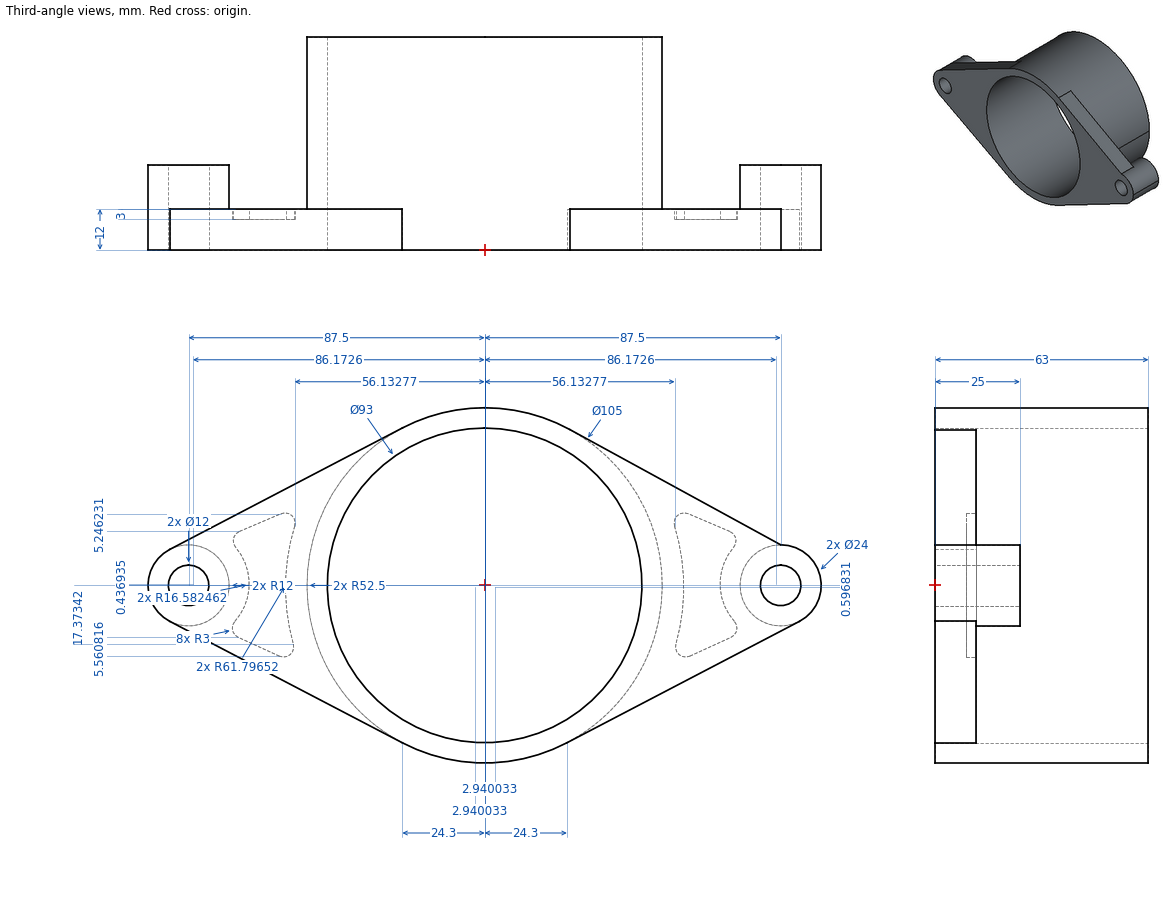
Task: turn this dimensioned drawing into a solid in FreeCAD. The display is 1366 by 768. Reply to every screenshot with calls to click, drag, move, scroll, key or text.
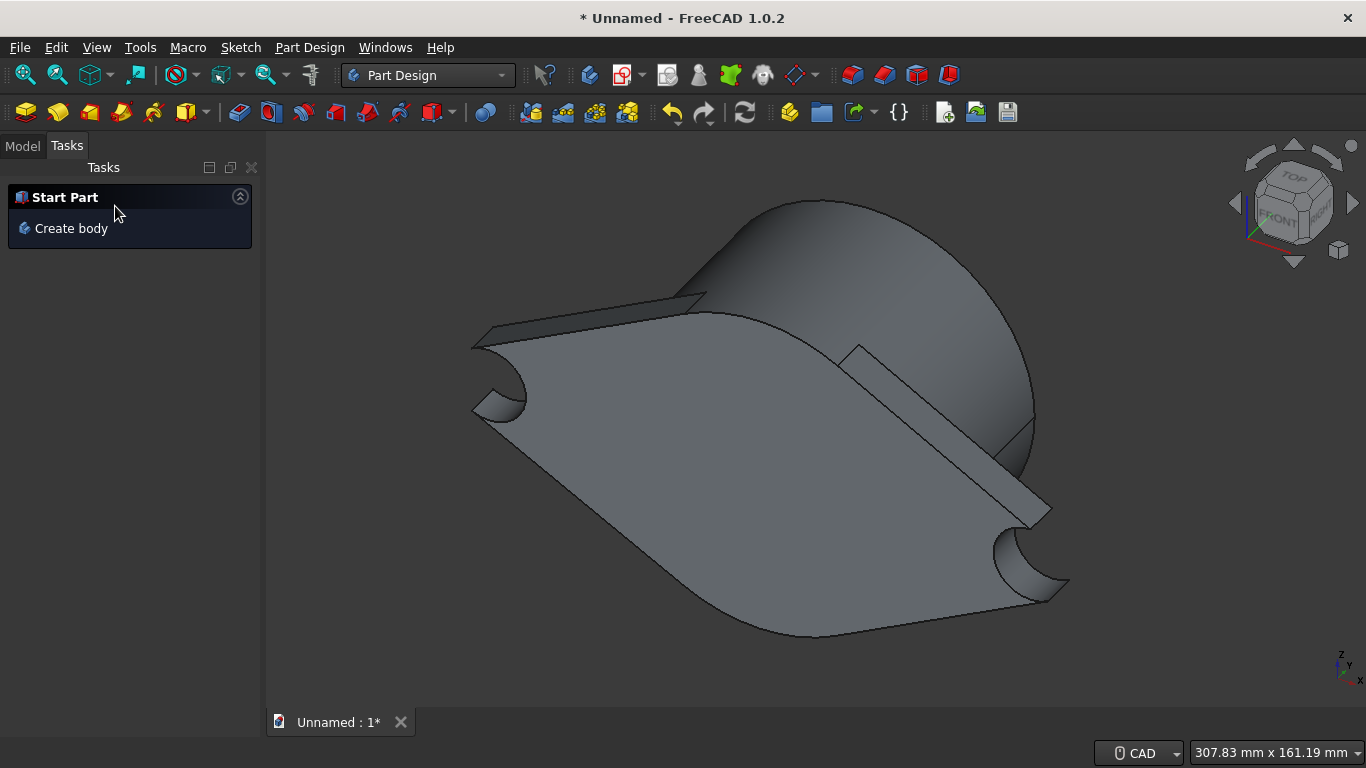
key(v)
key(f)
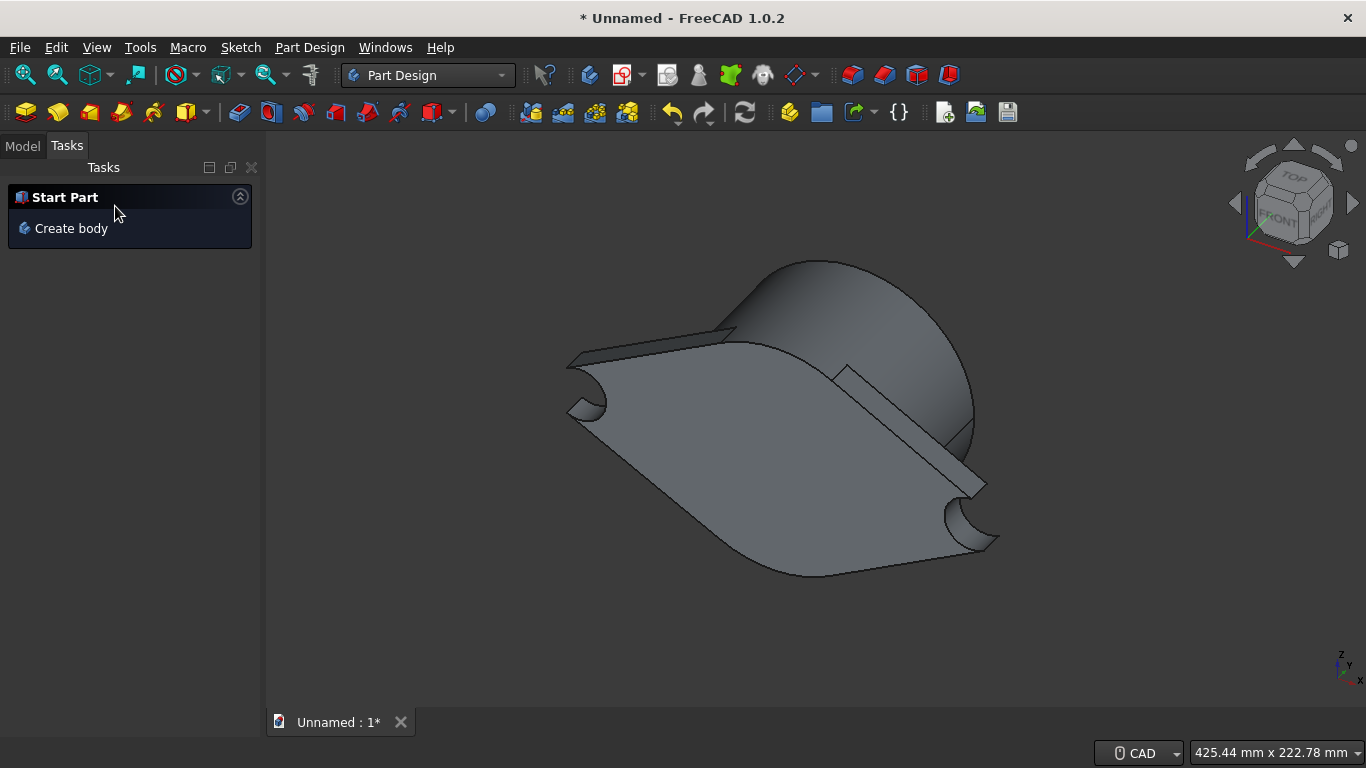
click(775, 458)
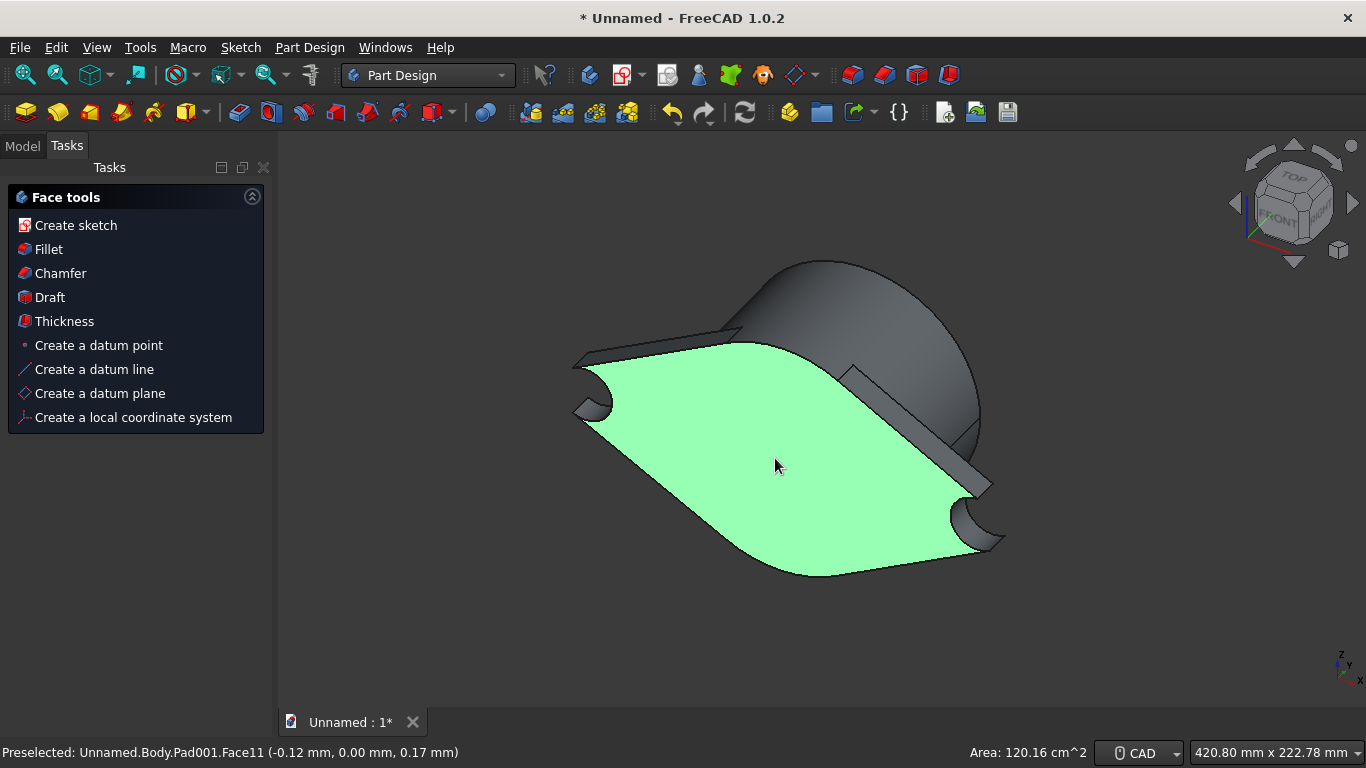
click(622, 76)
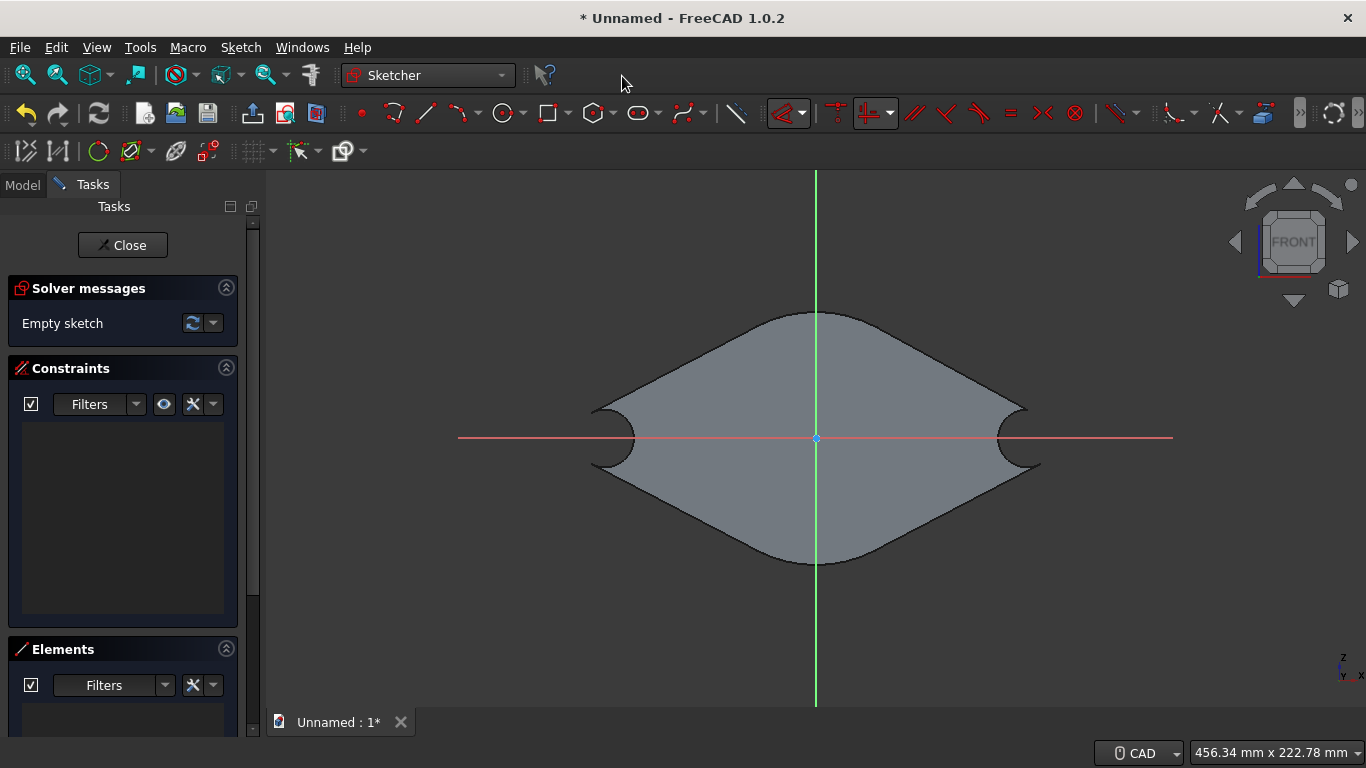
key(g)
key(c)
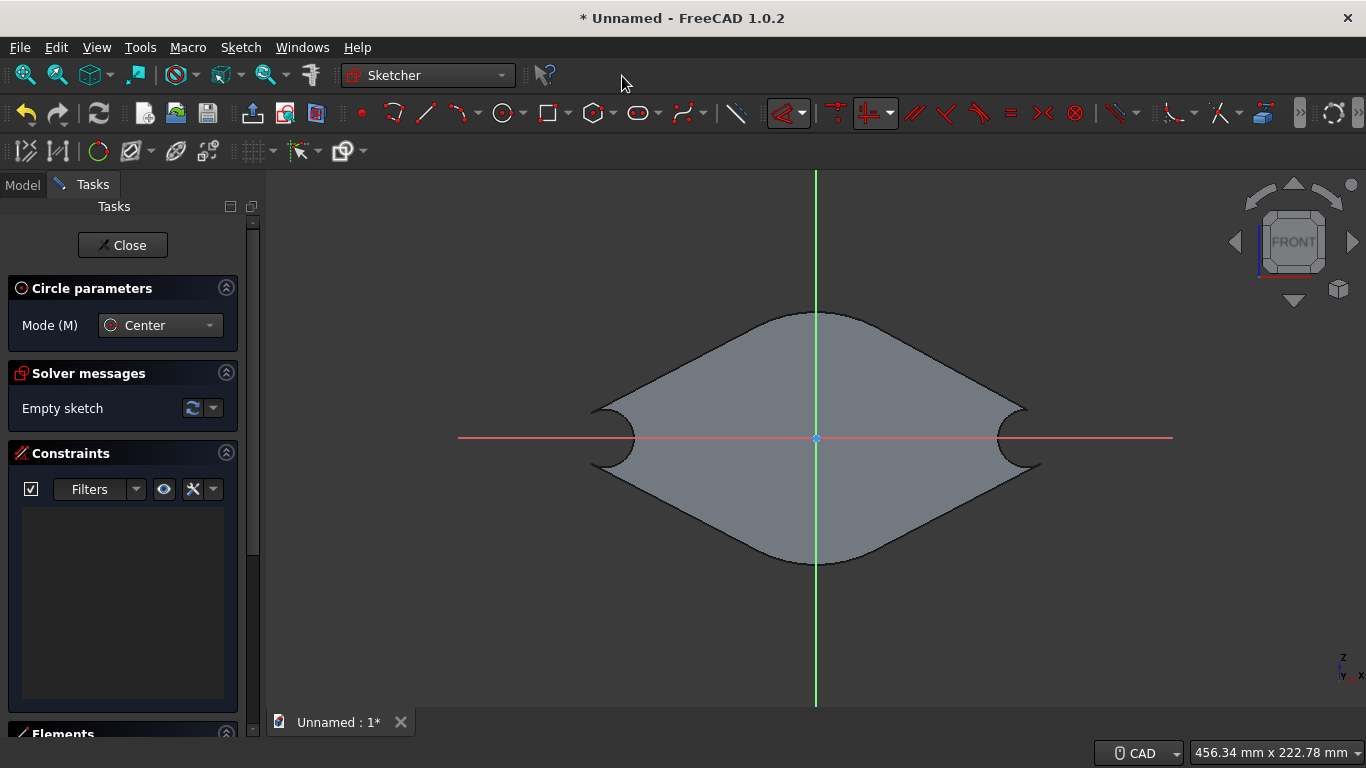
click(1027, 438)
move(1047, 418)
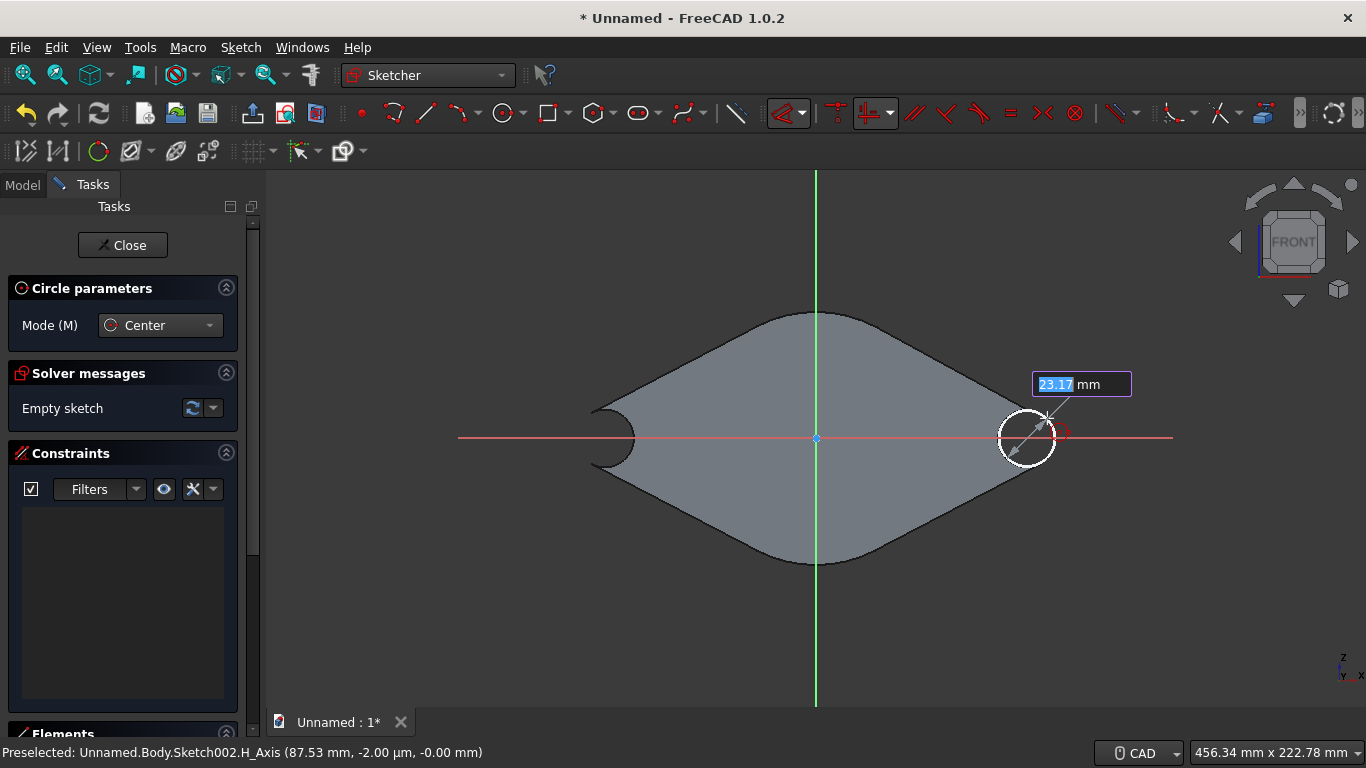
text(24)
key(Return)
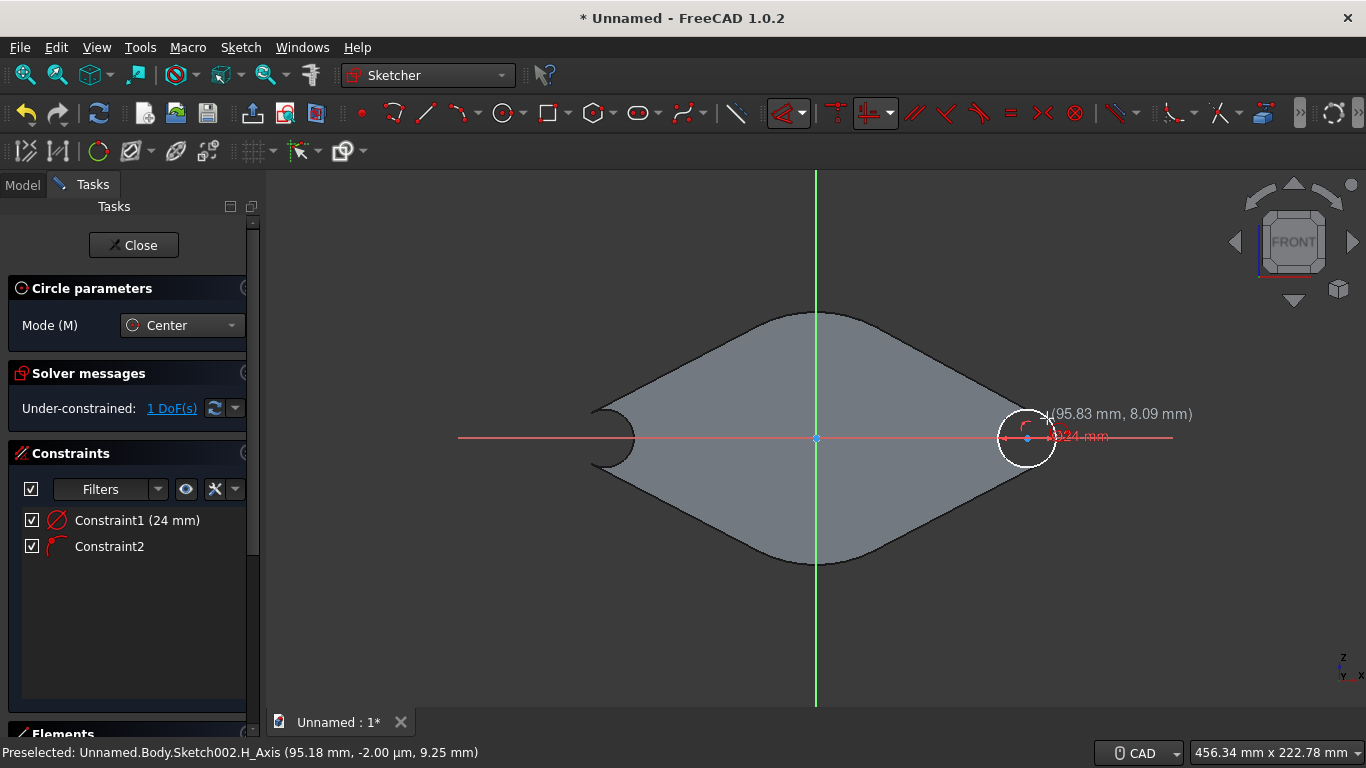
click(605, 438)
move(626, 418)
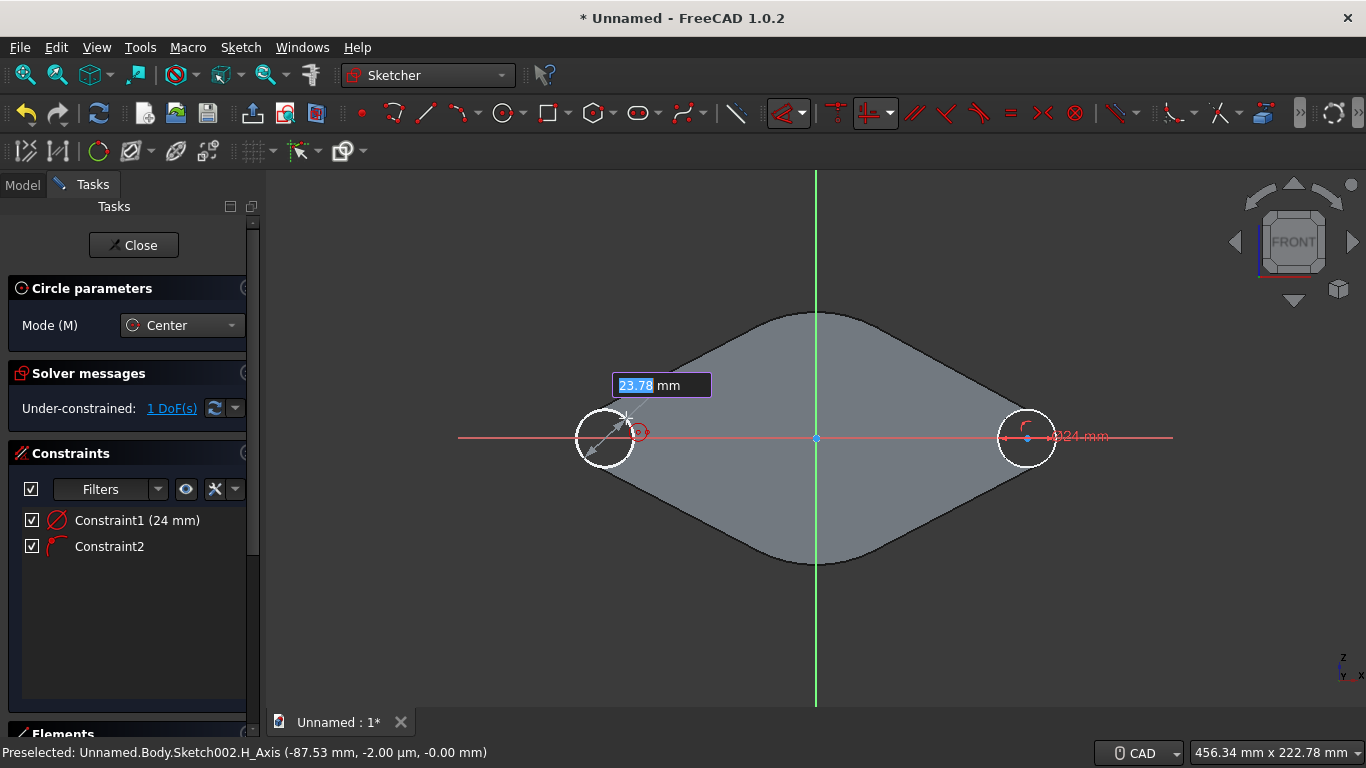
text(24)
key(Return)
key(Escape)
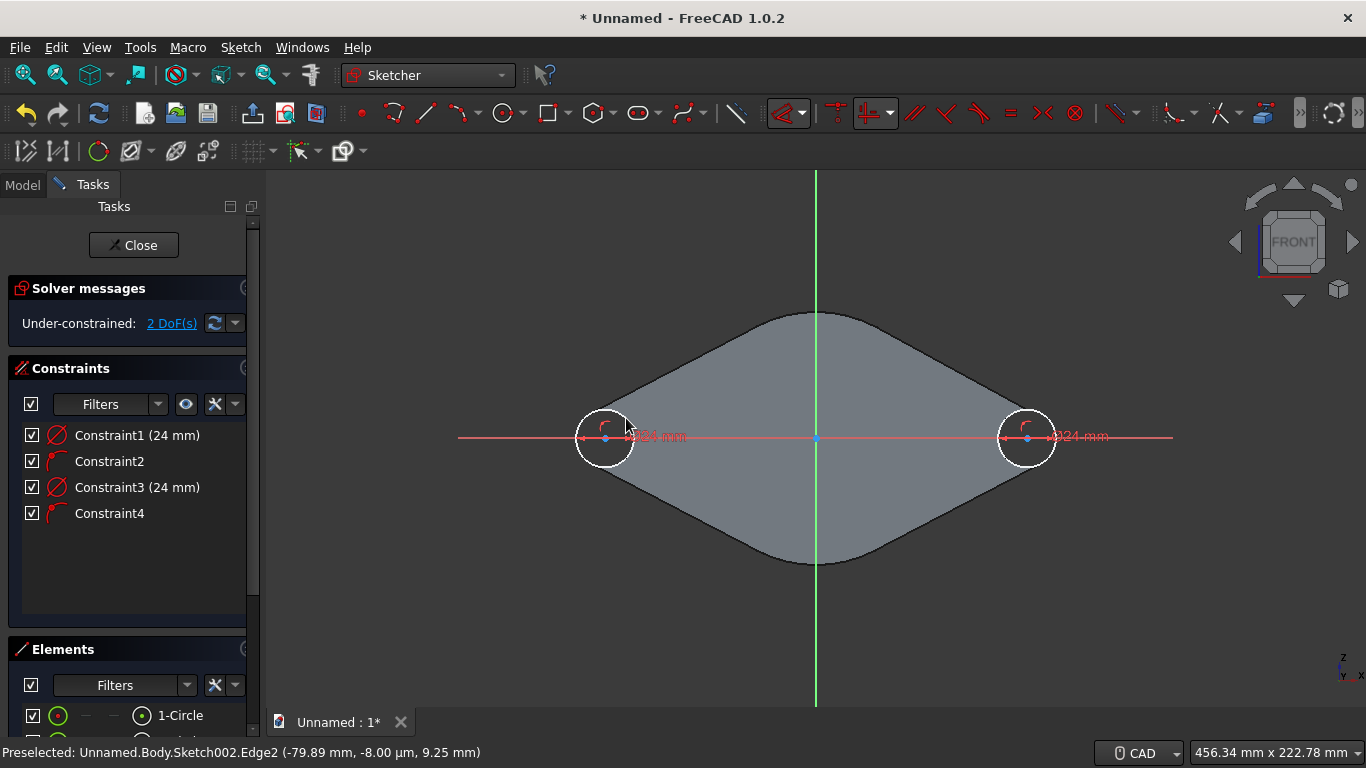
click(782, 114)